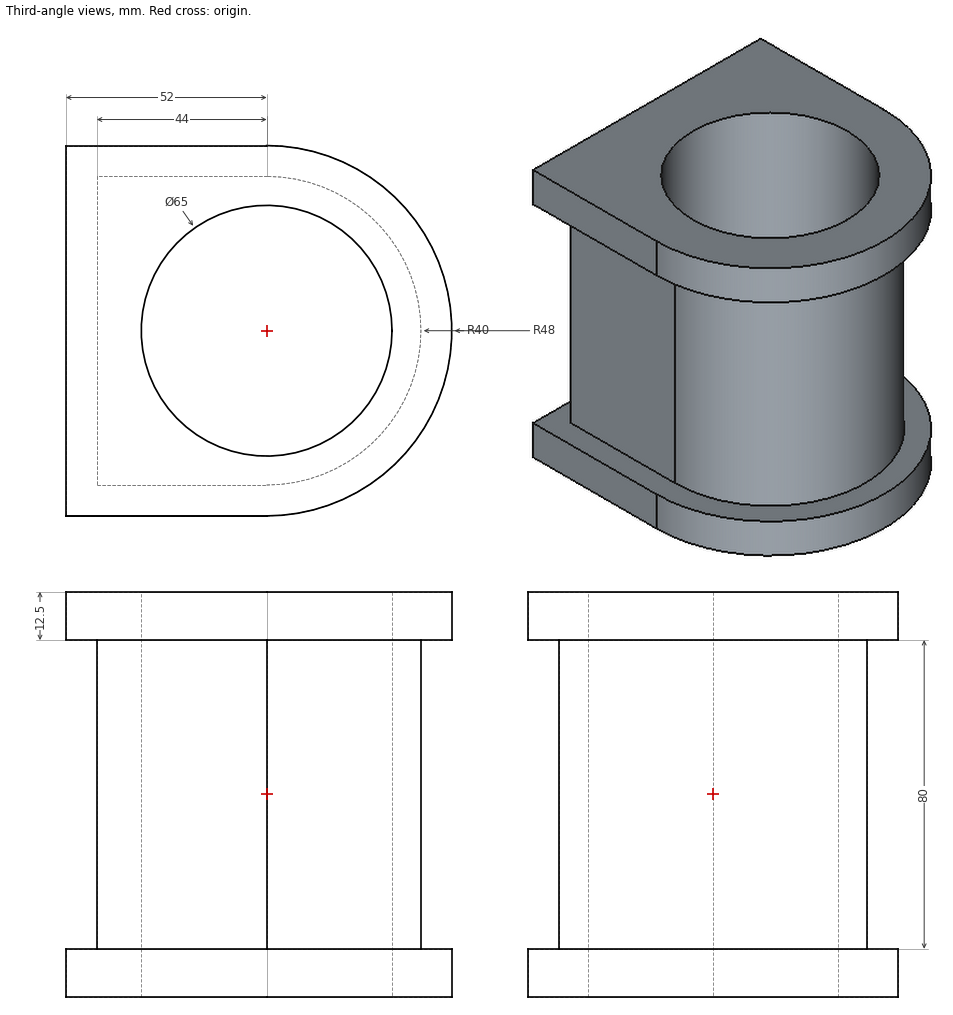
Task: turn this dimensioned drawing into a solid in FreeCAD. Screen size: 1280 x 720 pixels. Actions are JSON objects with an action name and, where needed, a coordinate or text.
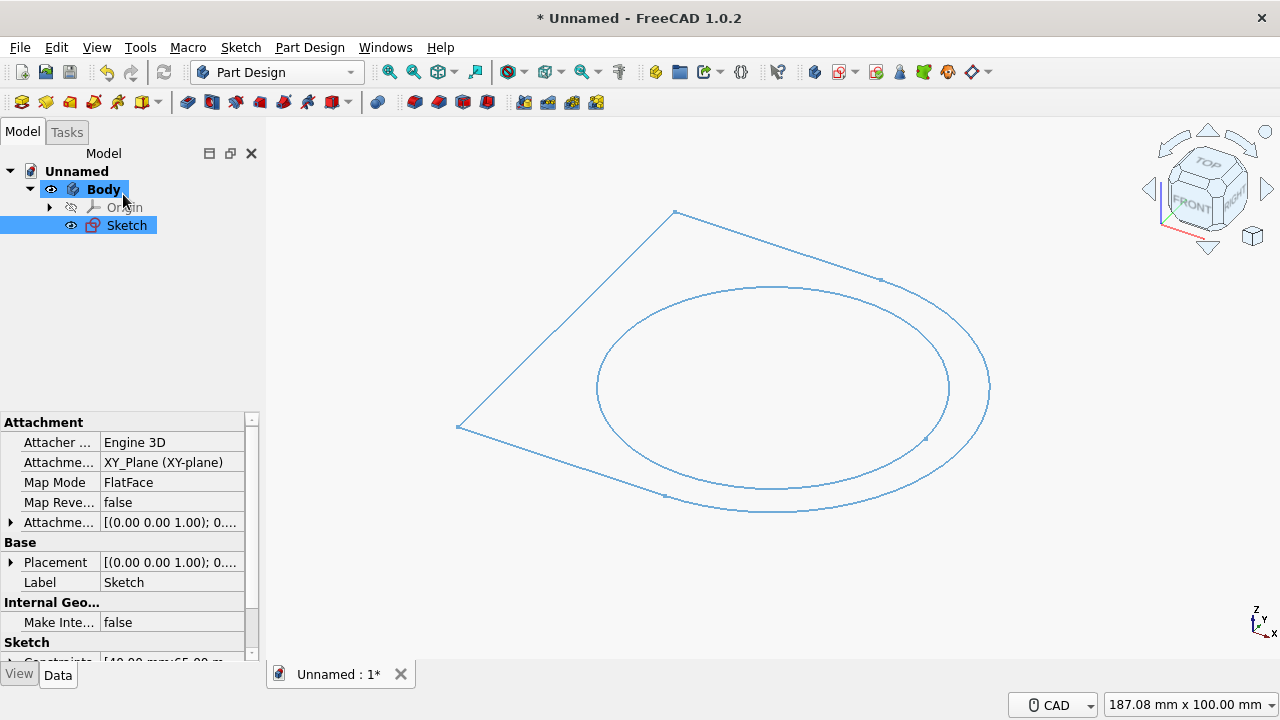
{"action": "left_click", "coordinate": [22, 102]}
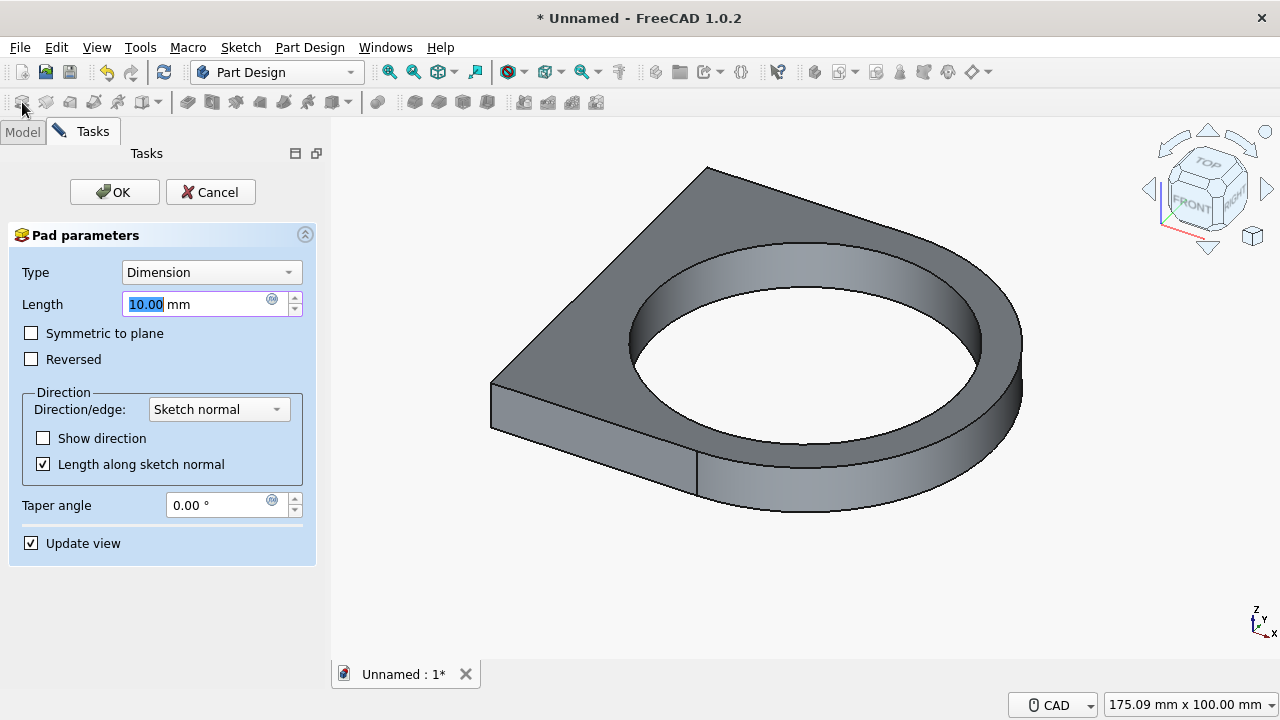
{"action": "type", "text": "80"}
{"action": "key", "text": "Tab"}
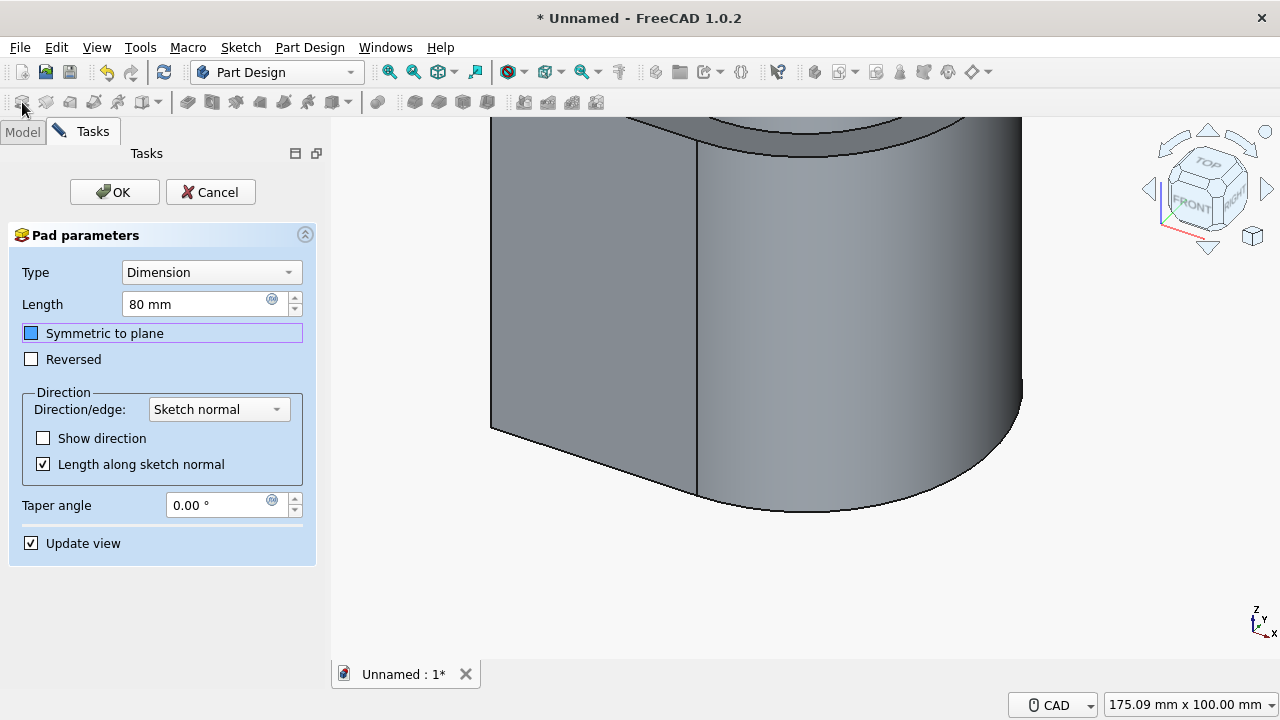
{"action": "left_click", "coordinate": [30, 333]}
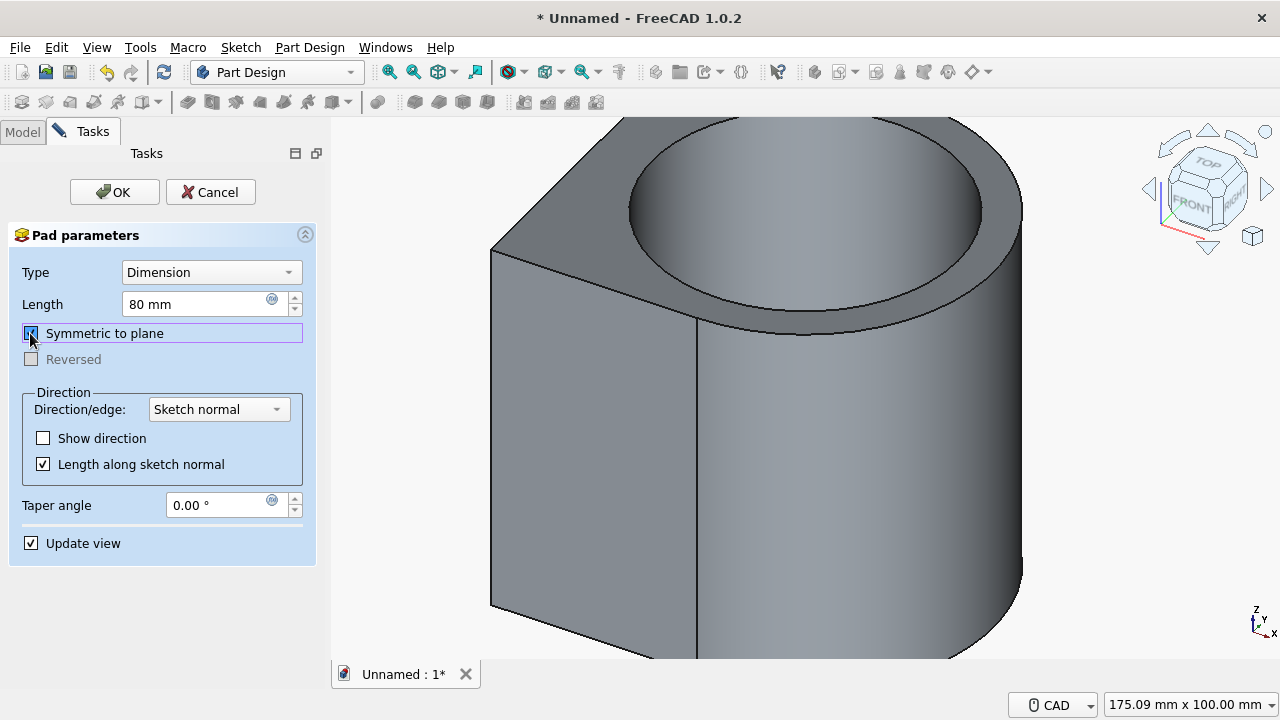
{"action": "left_click", "coordinate": [115, 192]}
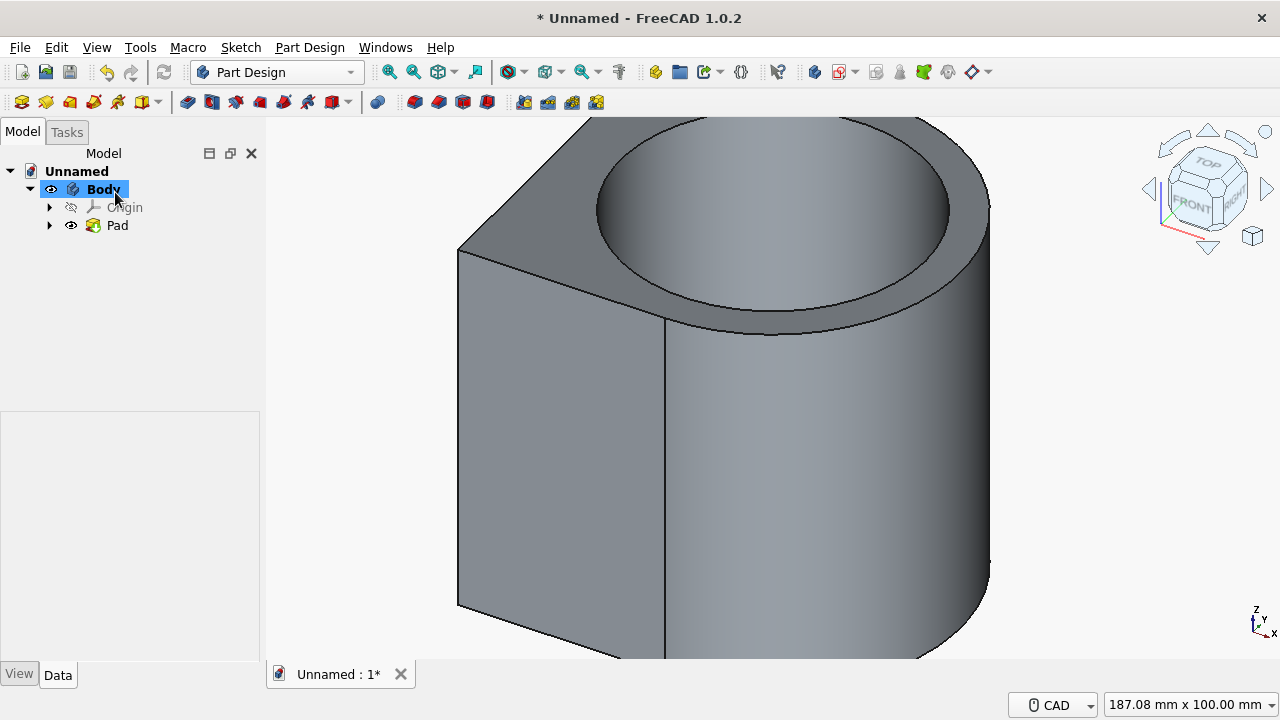
{"action": "left_click", "coordinate": [390, 72]}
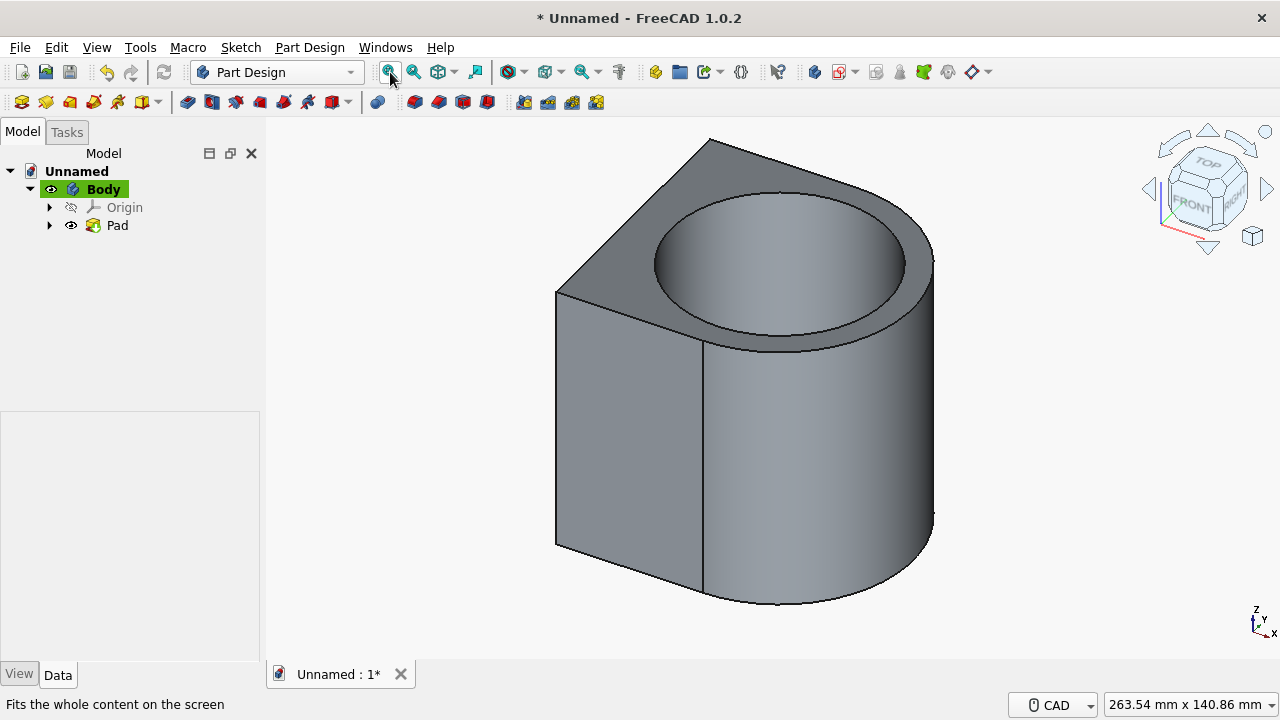
{"action": "left_click", "coordinate": [697, 178]}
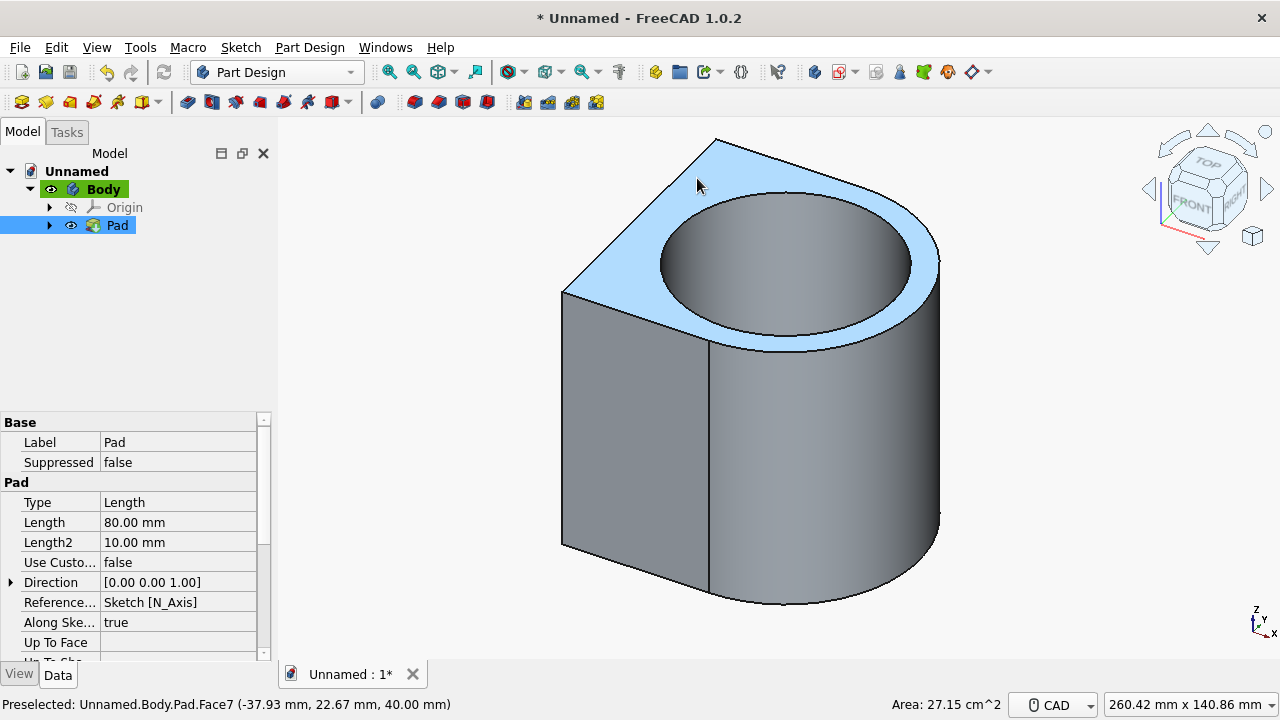
{"action": "left_click", "coordinate": [840, 72]}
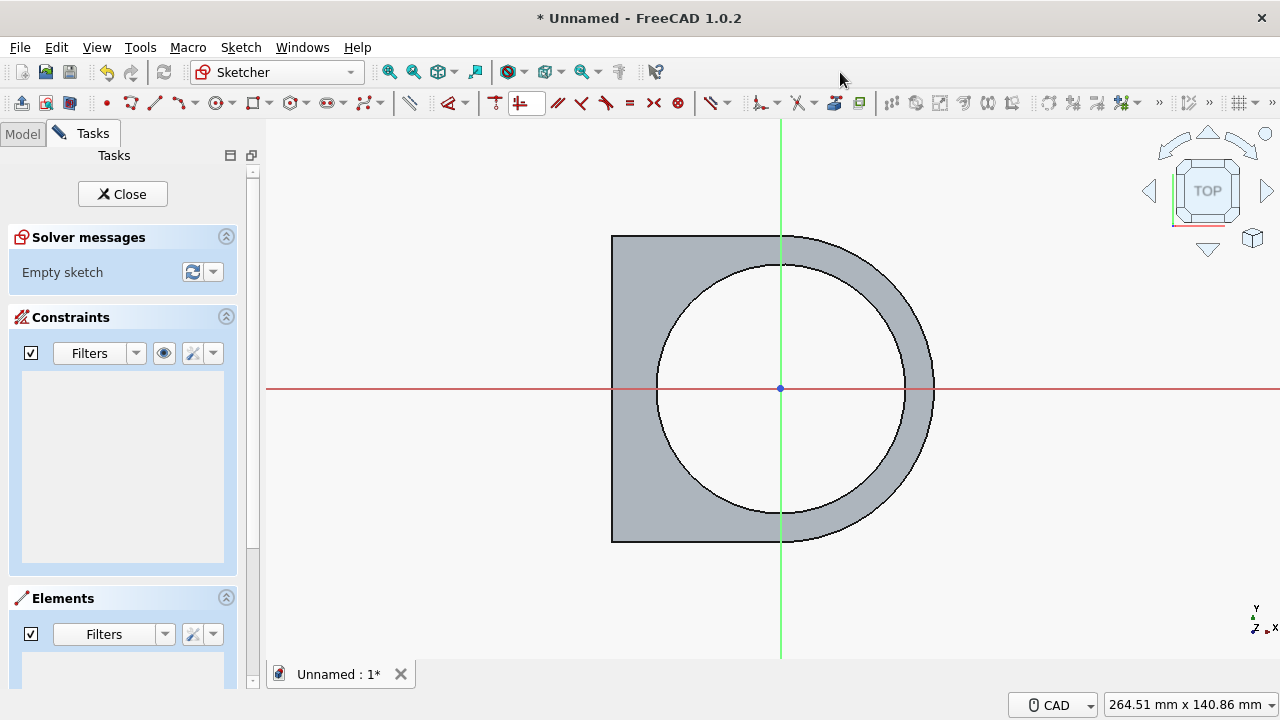
{"action": "left_click", "coordinate": [132, 104]}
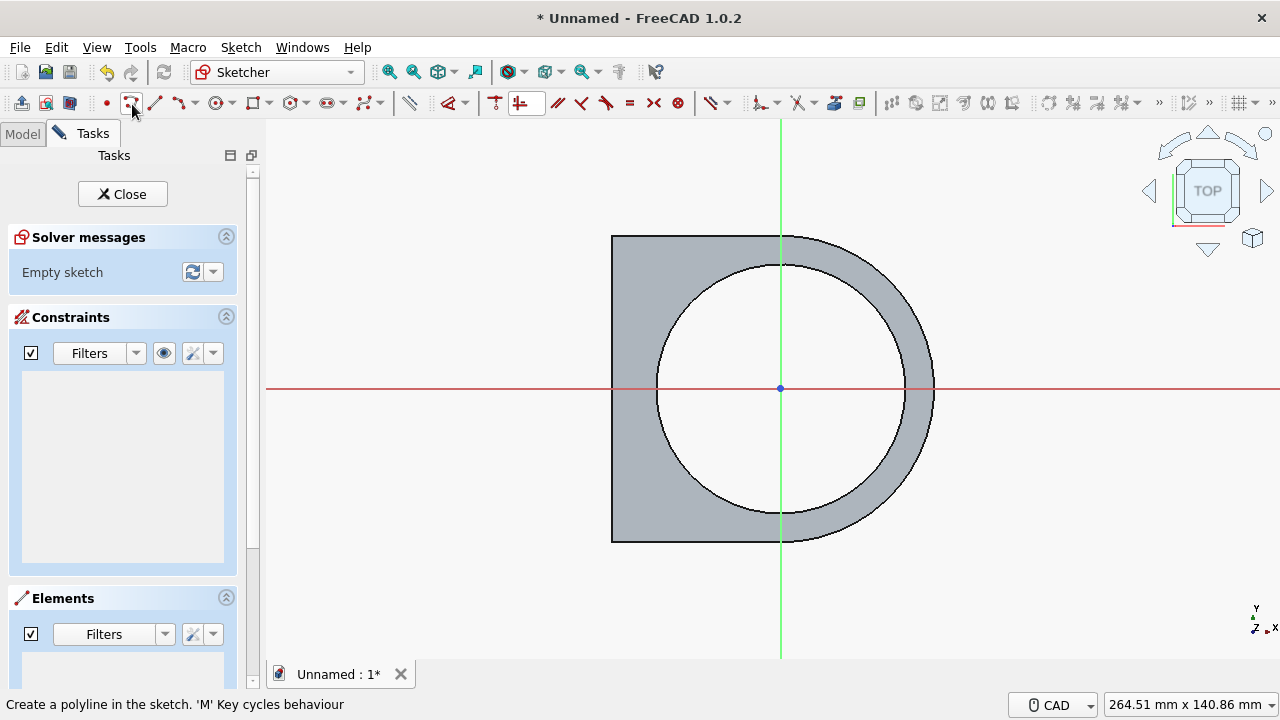
{"action": "left_click", "coordinate": [781, 205]}
{"action": "left_click", "coordinate": [581, 205]}
{"action": "left_click", "coordinate": [581, 573]}
{"action": "left_click", "coordinate": [781, 573]}
{"action": "right_click", "coordinate": [781, 573]}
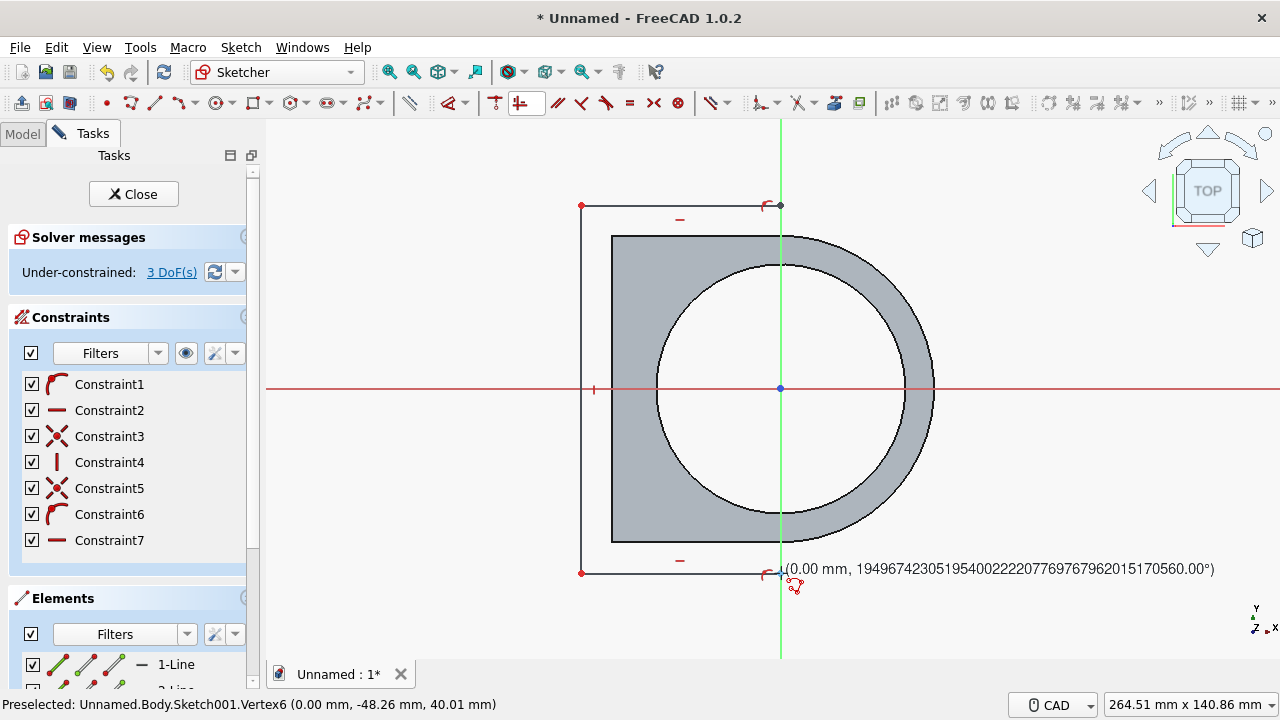
{"action": "left_click", "coordinate": [180, 104]}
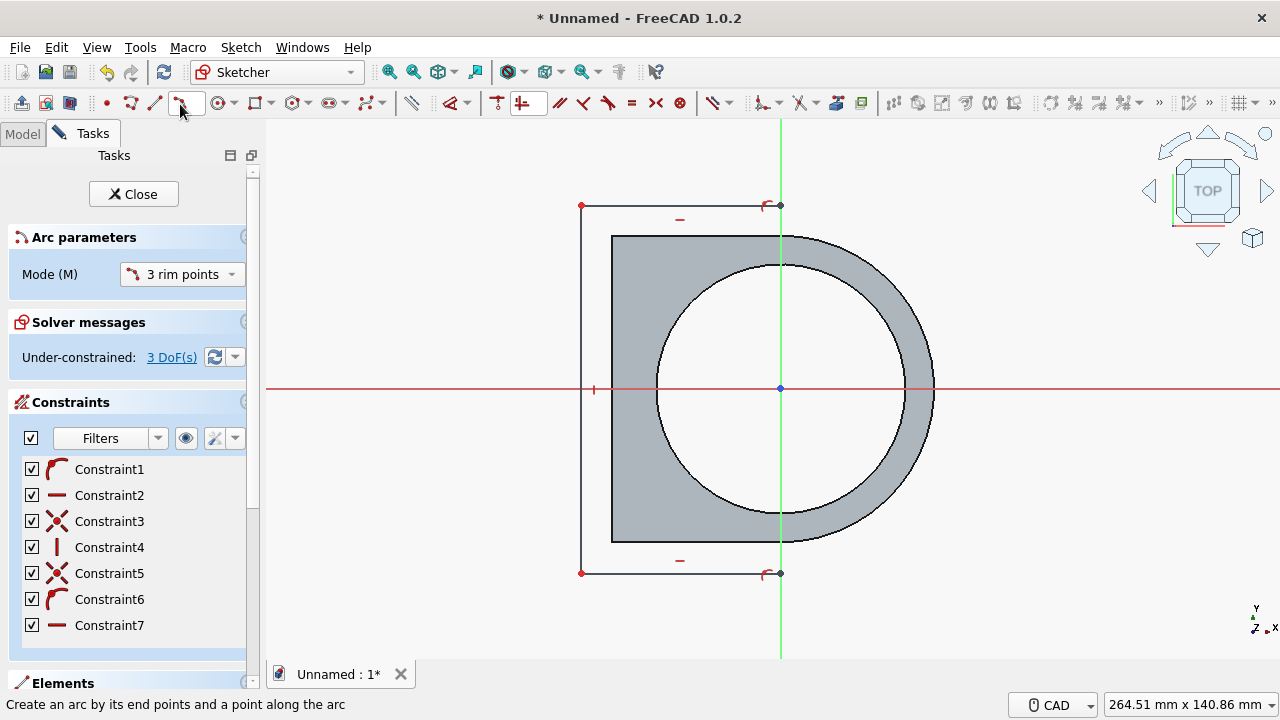
{"action": "left_click", "coordinate": [781, 574]}
{"action": "left_click", "coordinate": [781, 206]}
{"action": "left_click", "coordinate": [956, 446]}